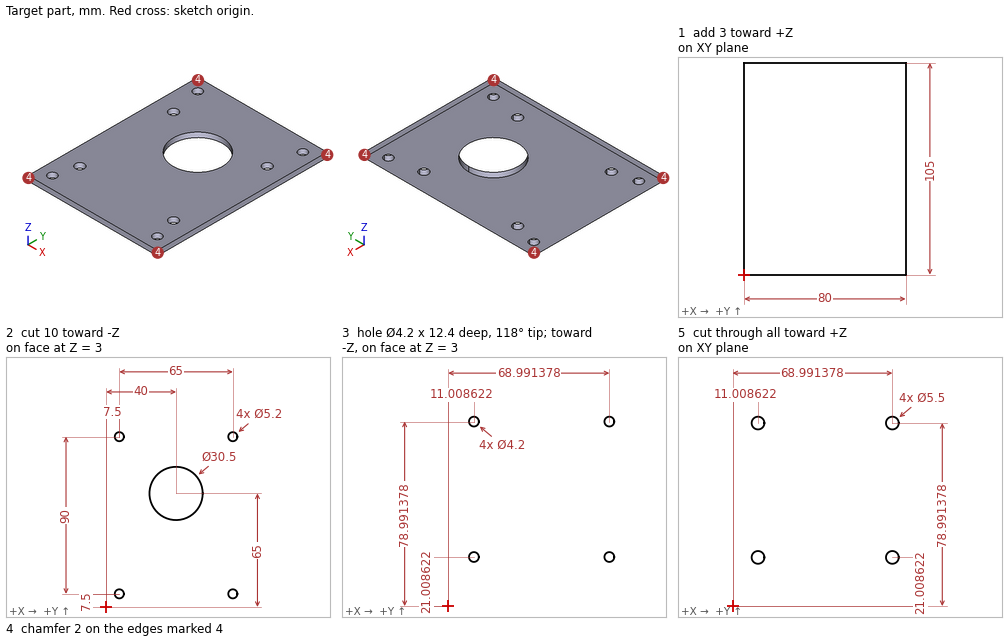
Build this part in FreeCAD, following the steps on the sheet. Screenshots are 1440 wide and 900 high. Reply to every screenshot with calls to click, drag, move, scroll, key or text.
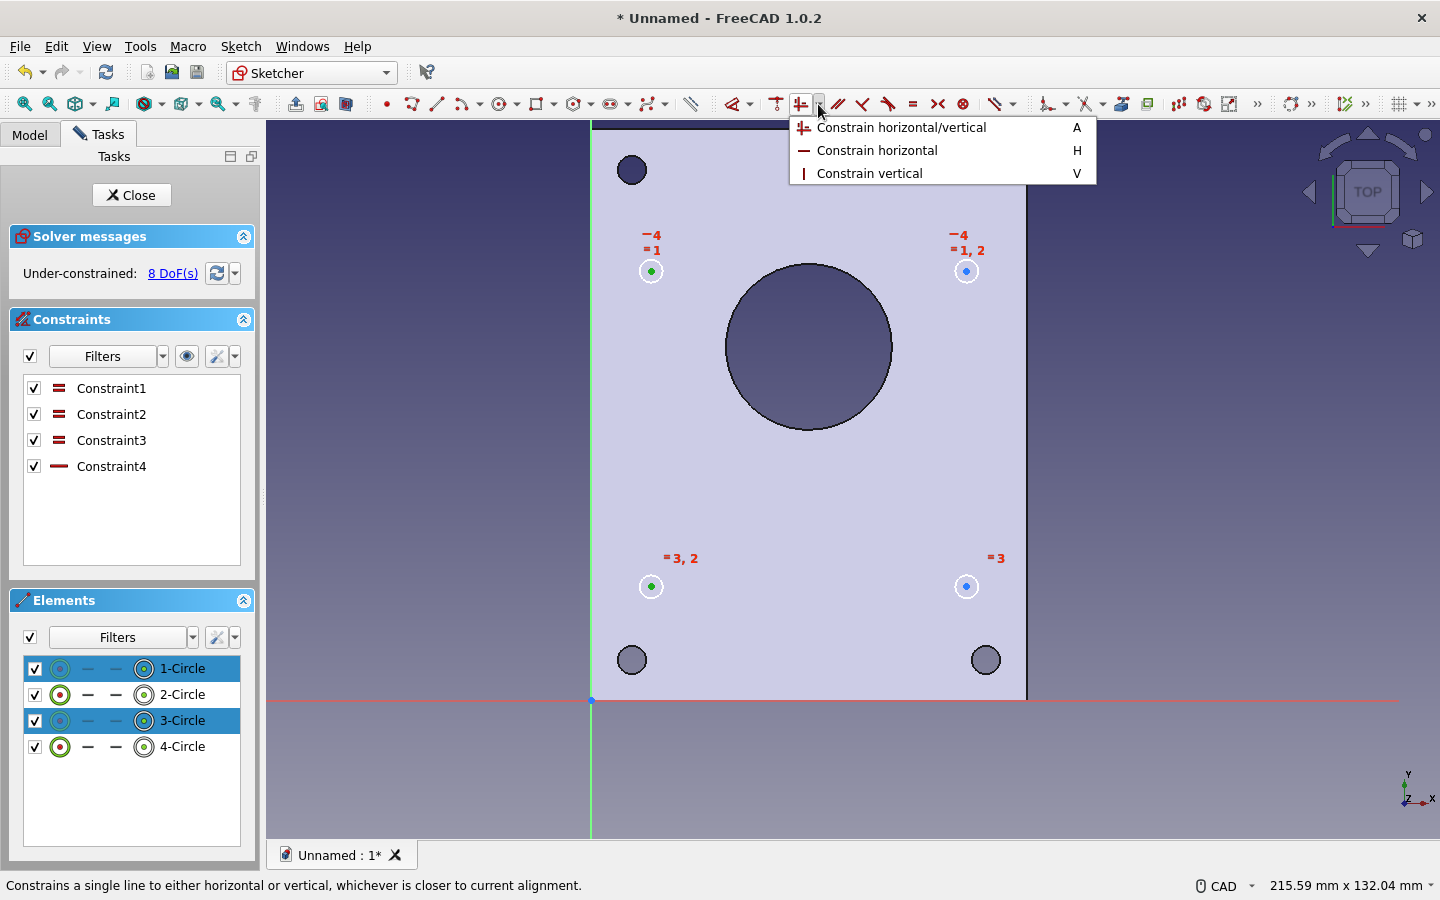
click(943, 174)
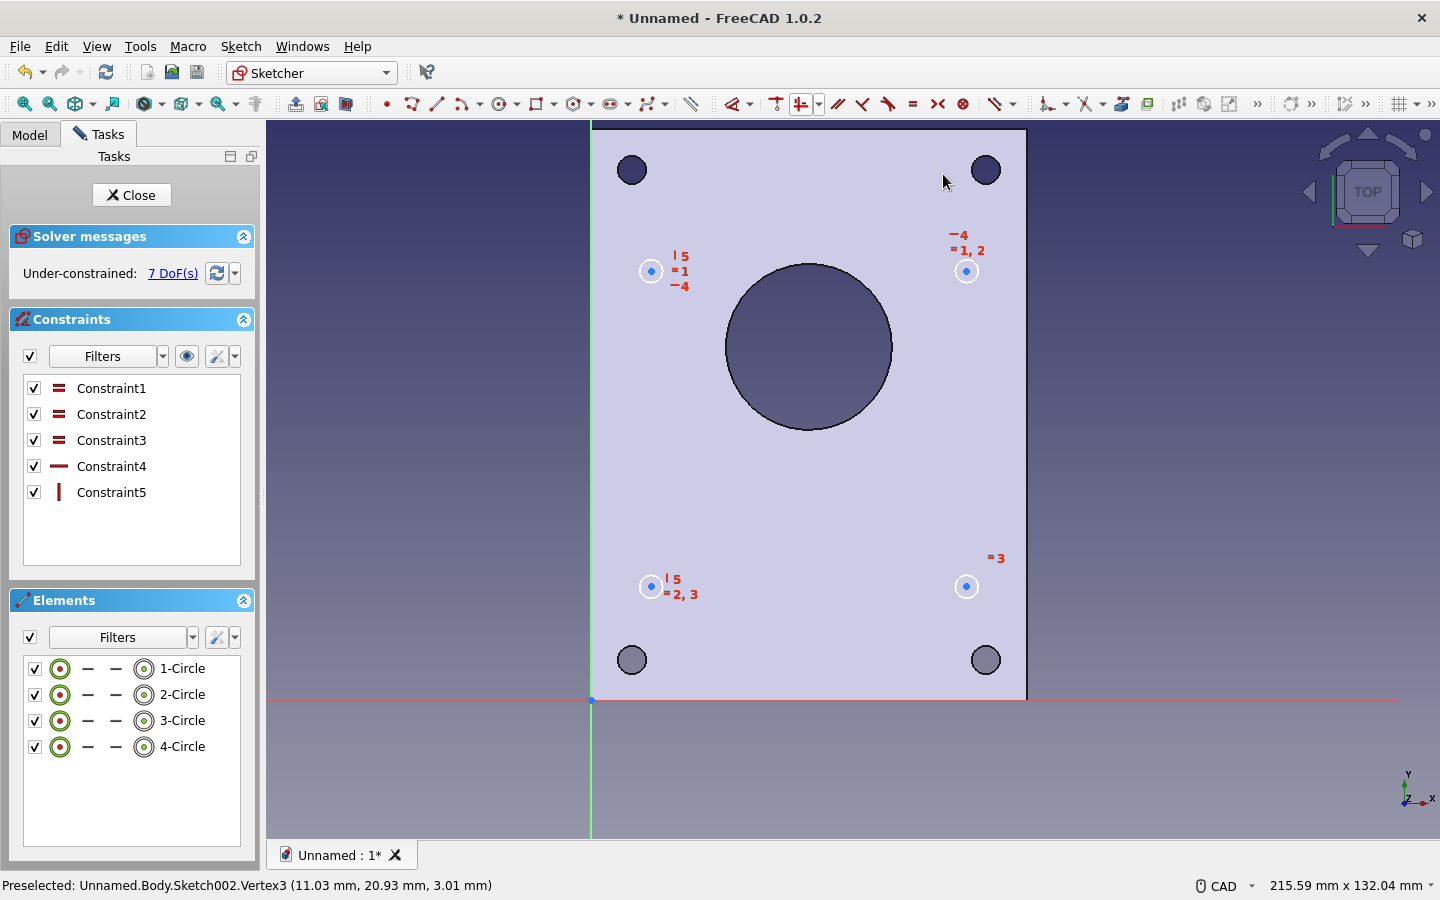
click(967, 271)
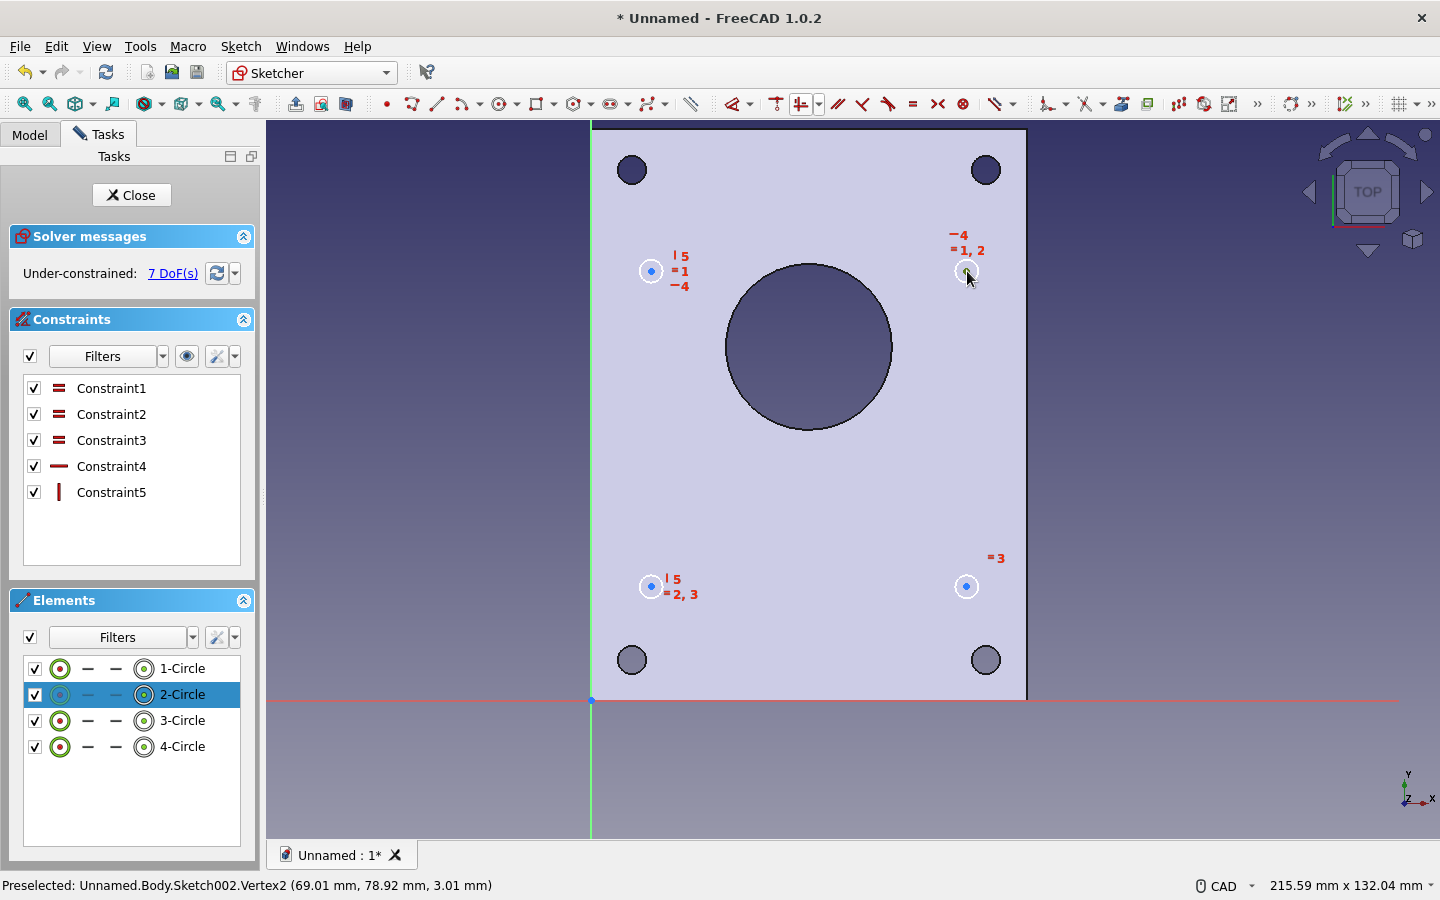
click(967, 587)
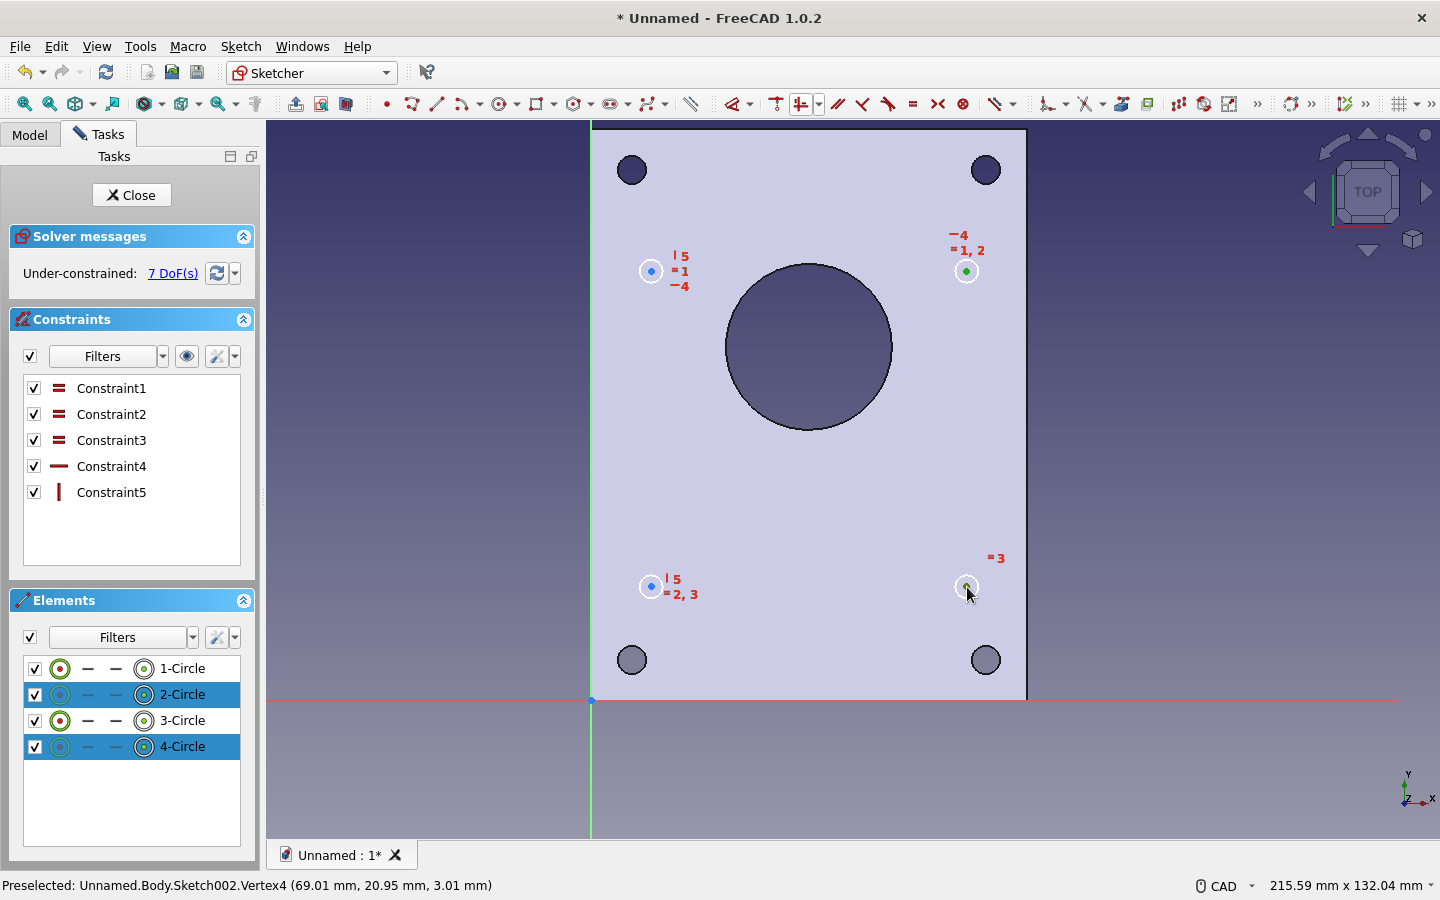
click(818, 104)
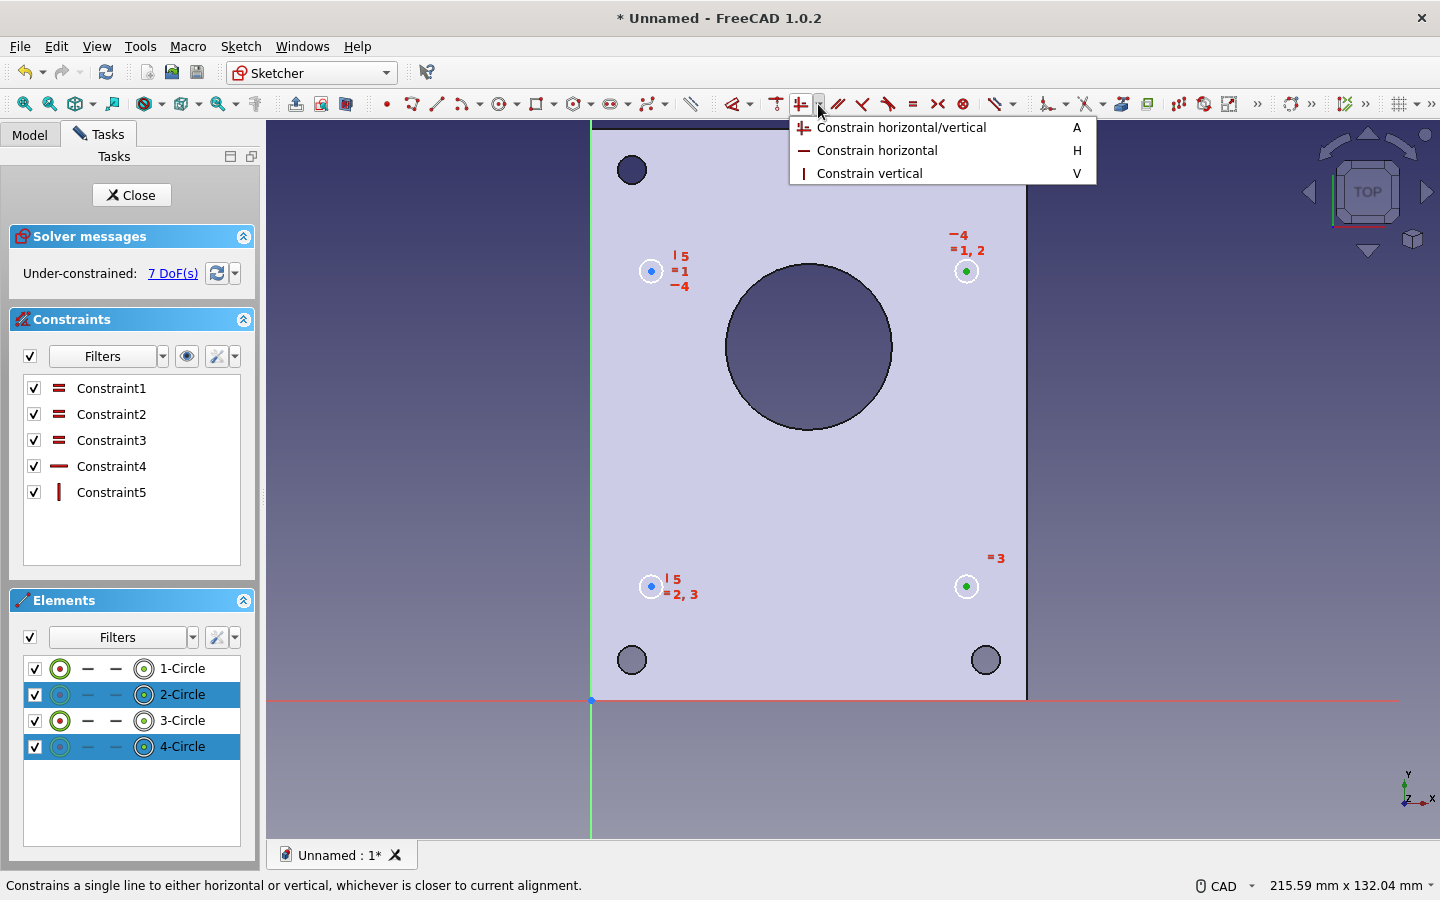
click(943, 174)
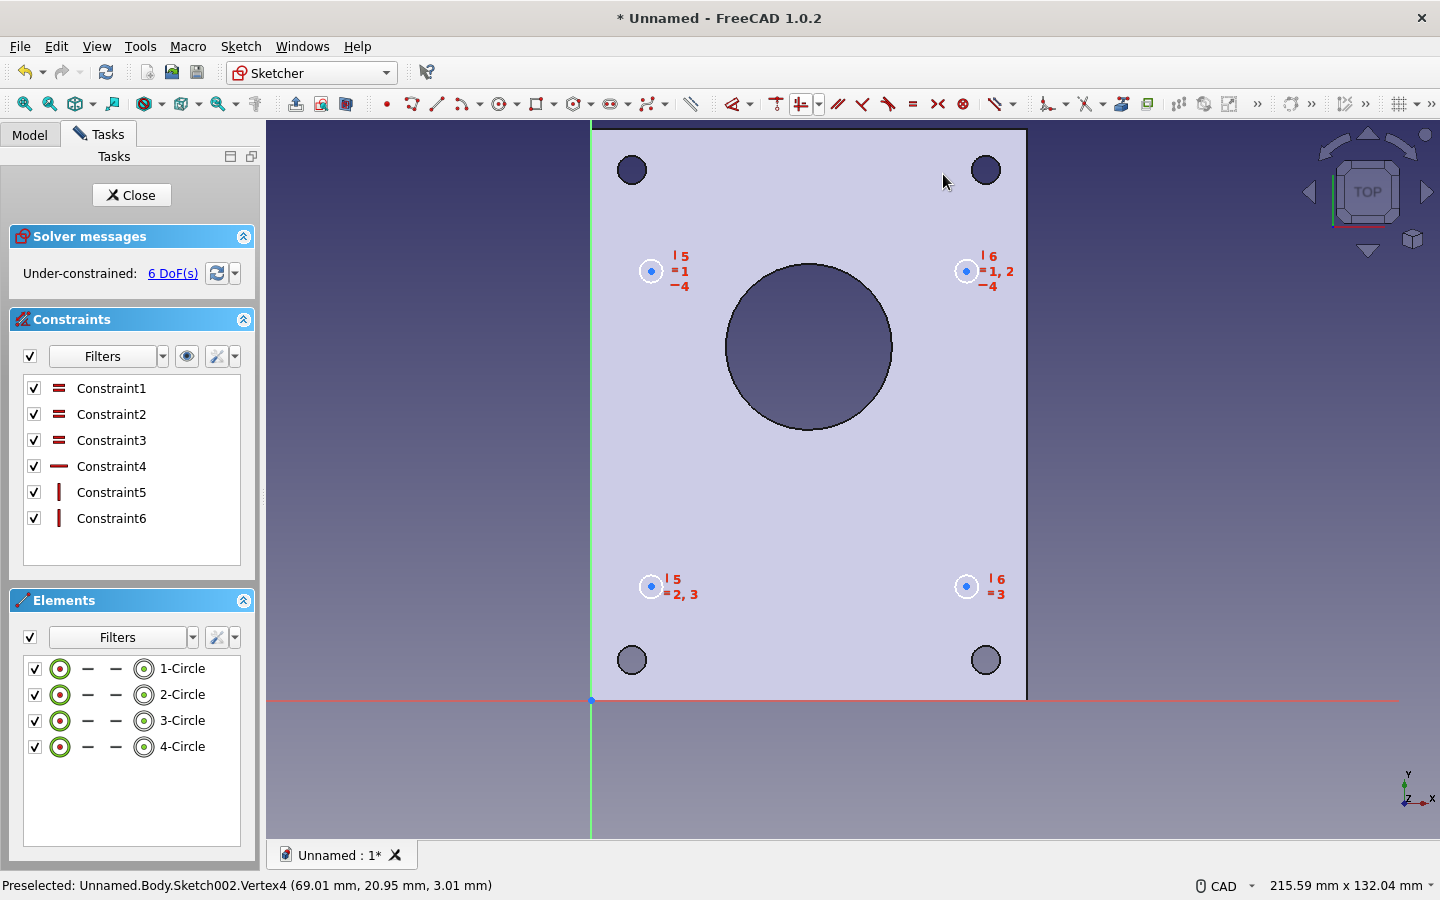
click(651, 587)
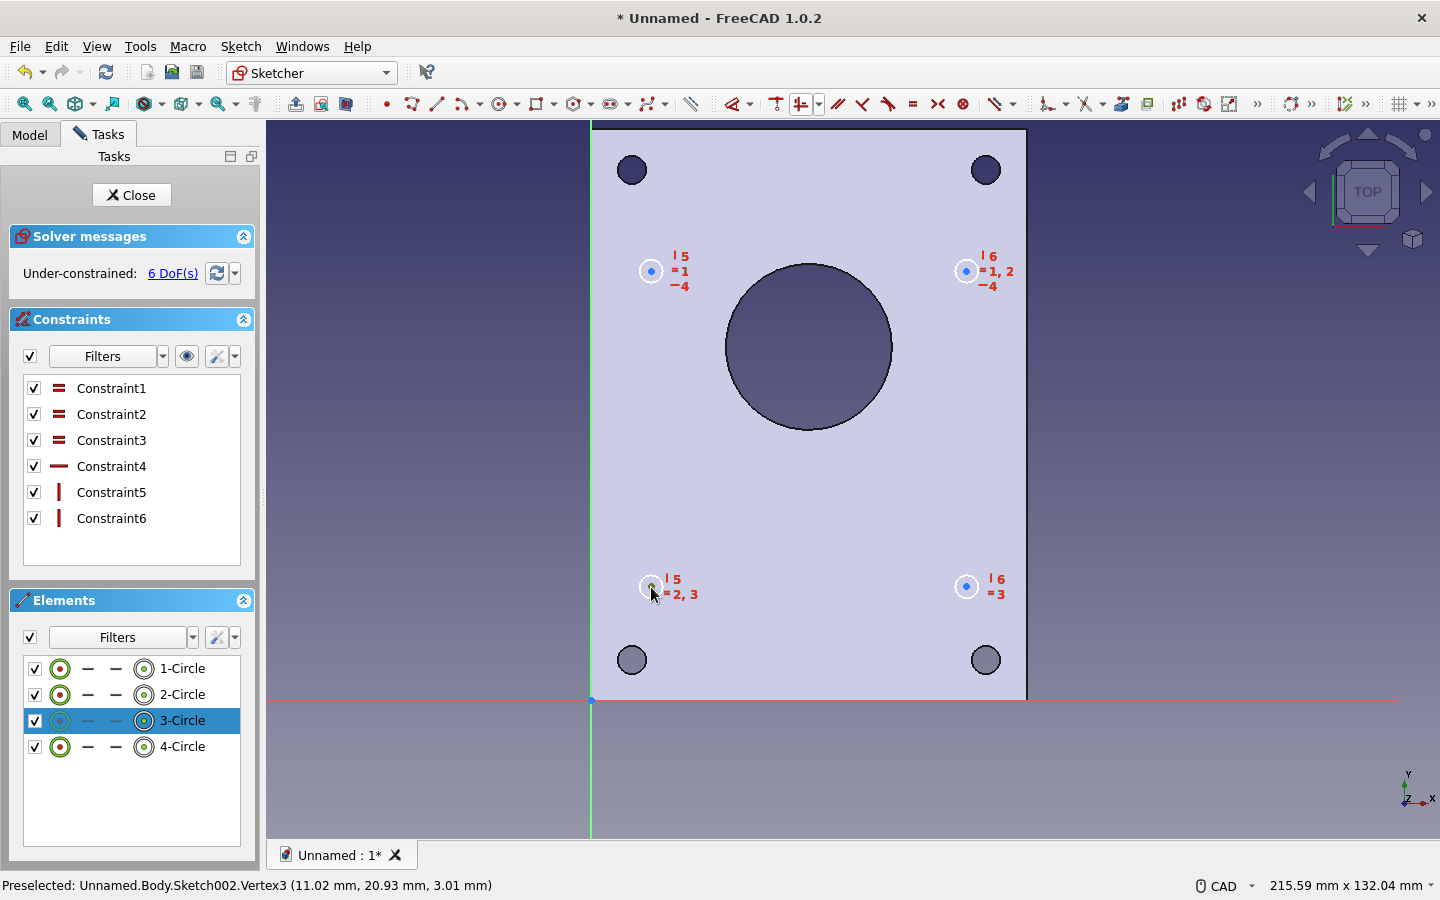
click(967, 587)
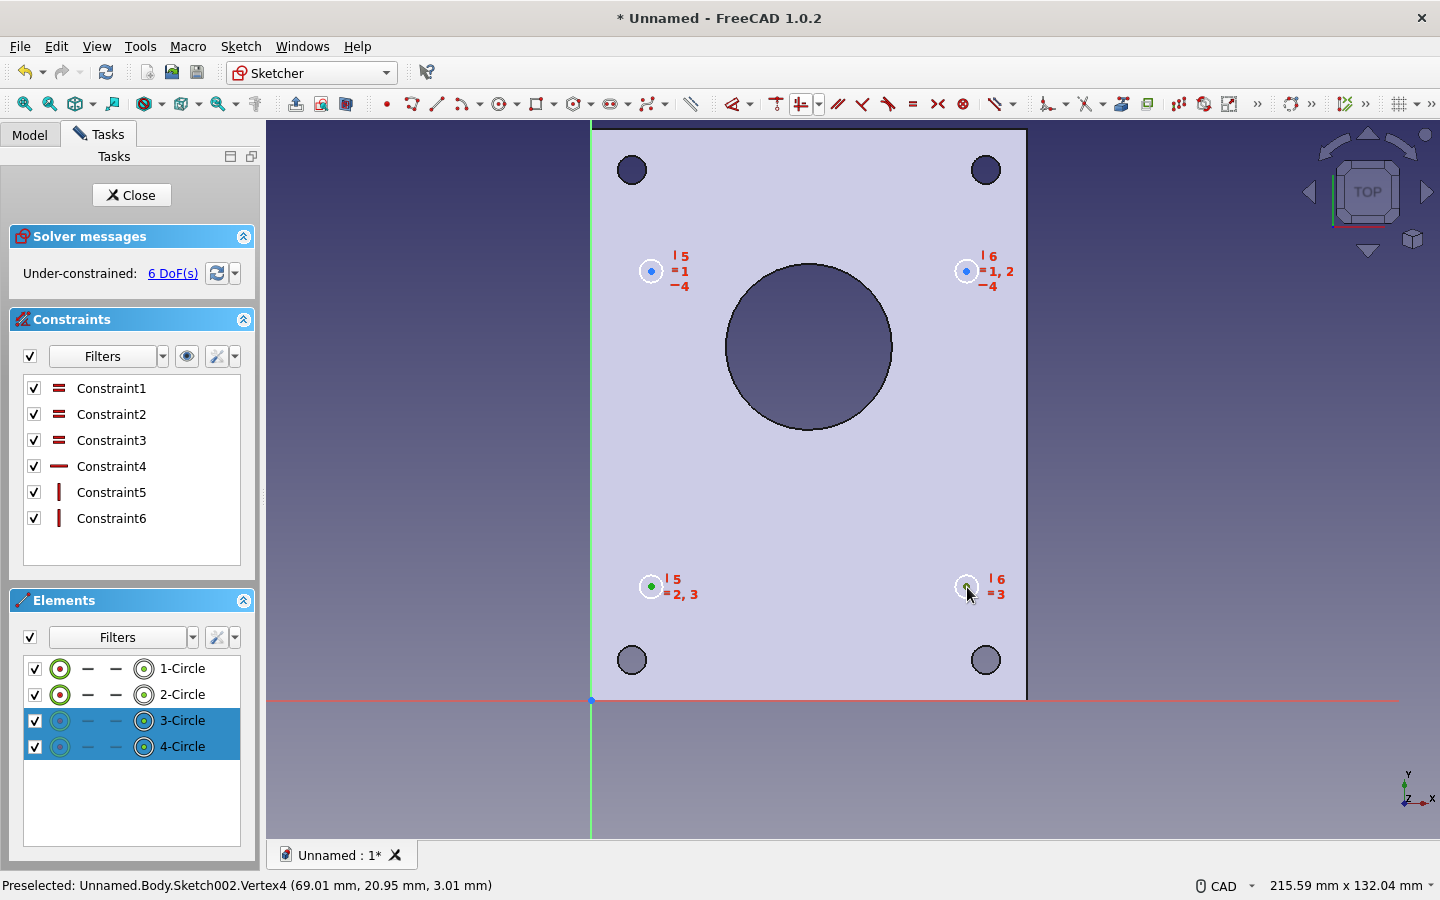
click(818, 104)